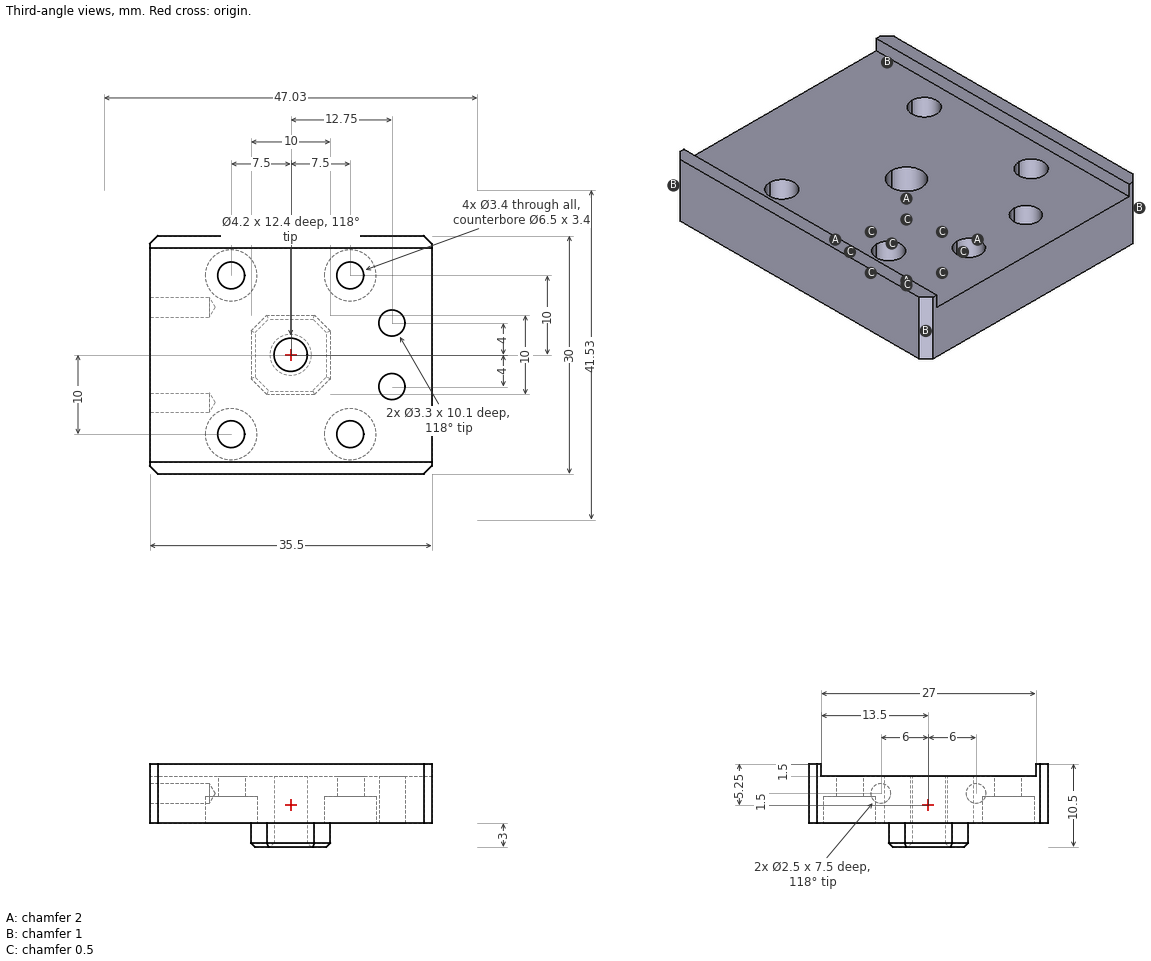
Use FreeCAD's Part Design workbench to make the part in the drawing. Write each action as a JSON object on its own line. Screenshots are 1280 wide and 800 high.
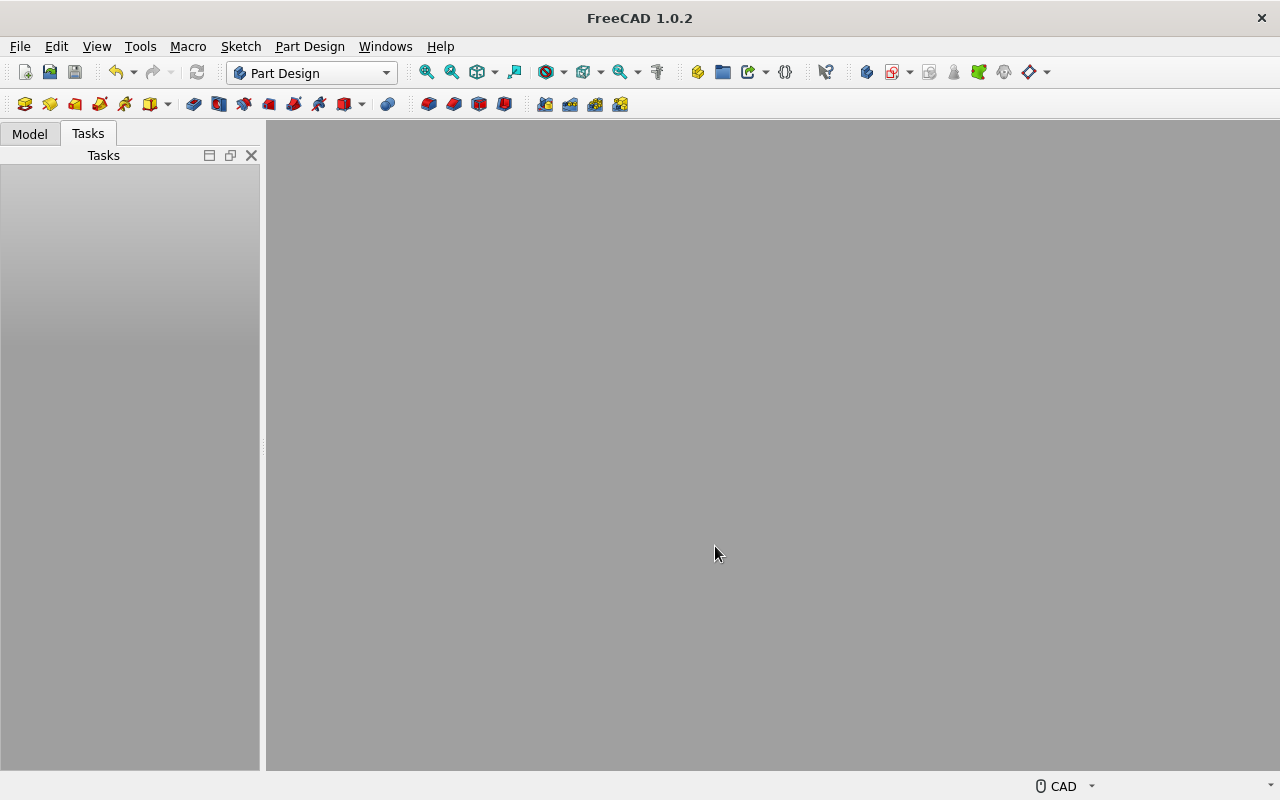
{"action": "key", "text": "ctrl+n"}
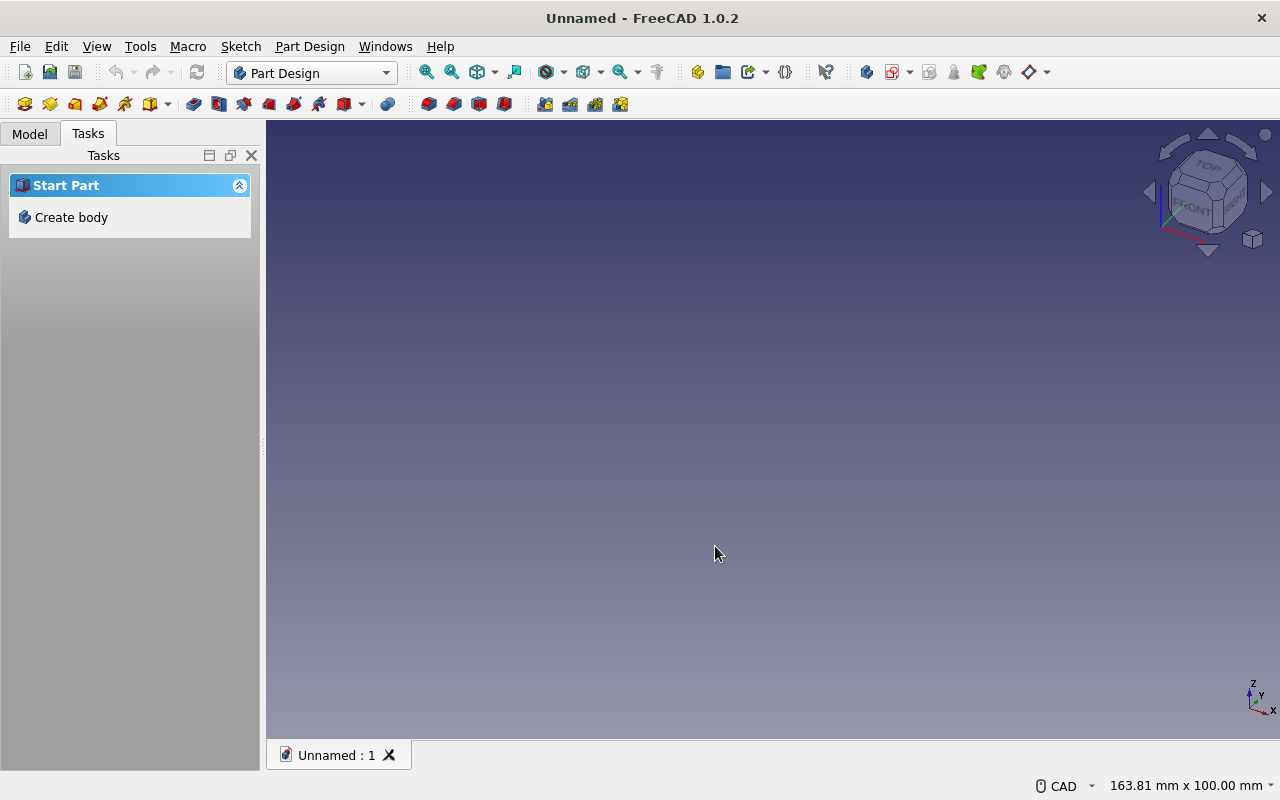
{"action": "left_click", "coordinate": [892, 72]}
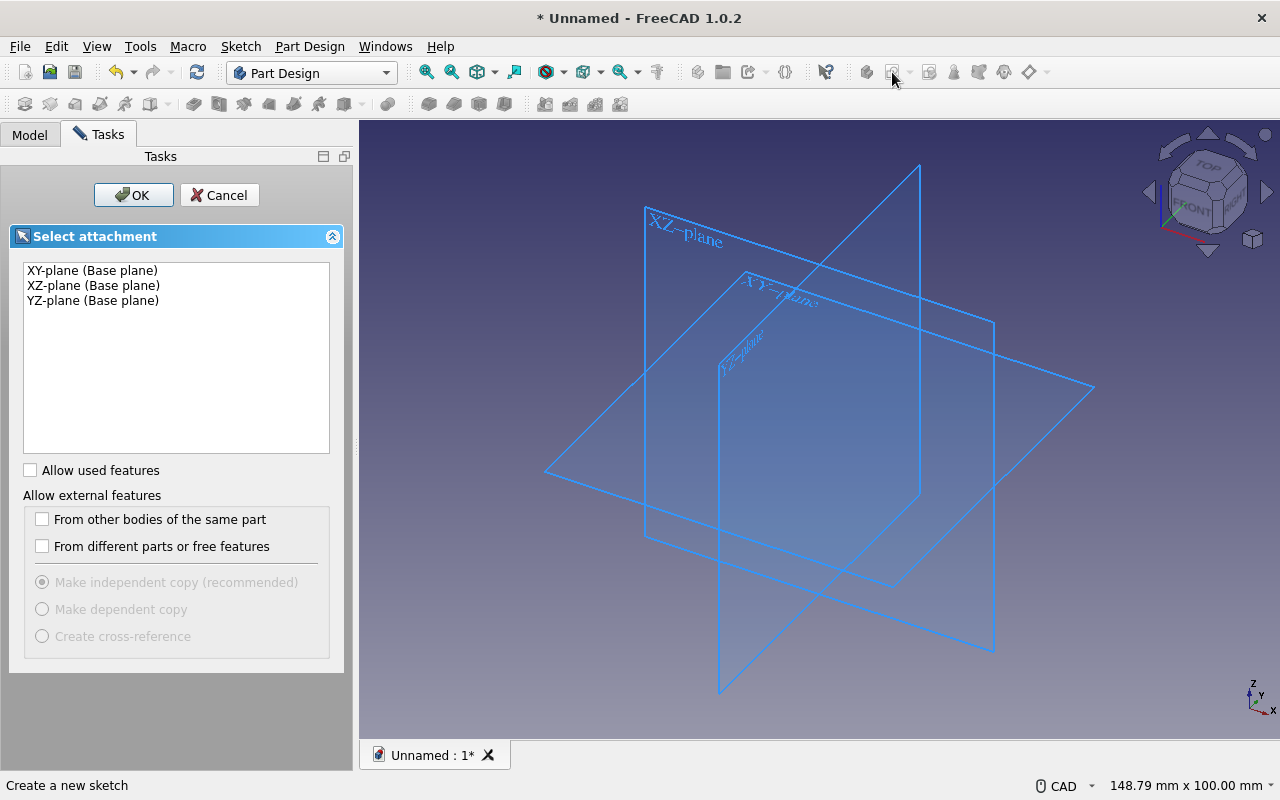
{"action": "left_click", "coordinate": [84, 270]}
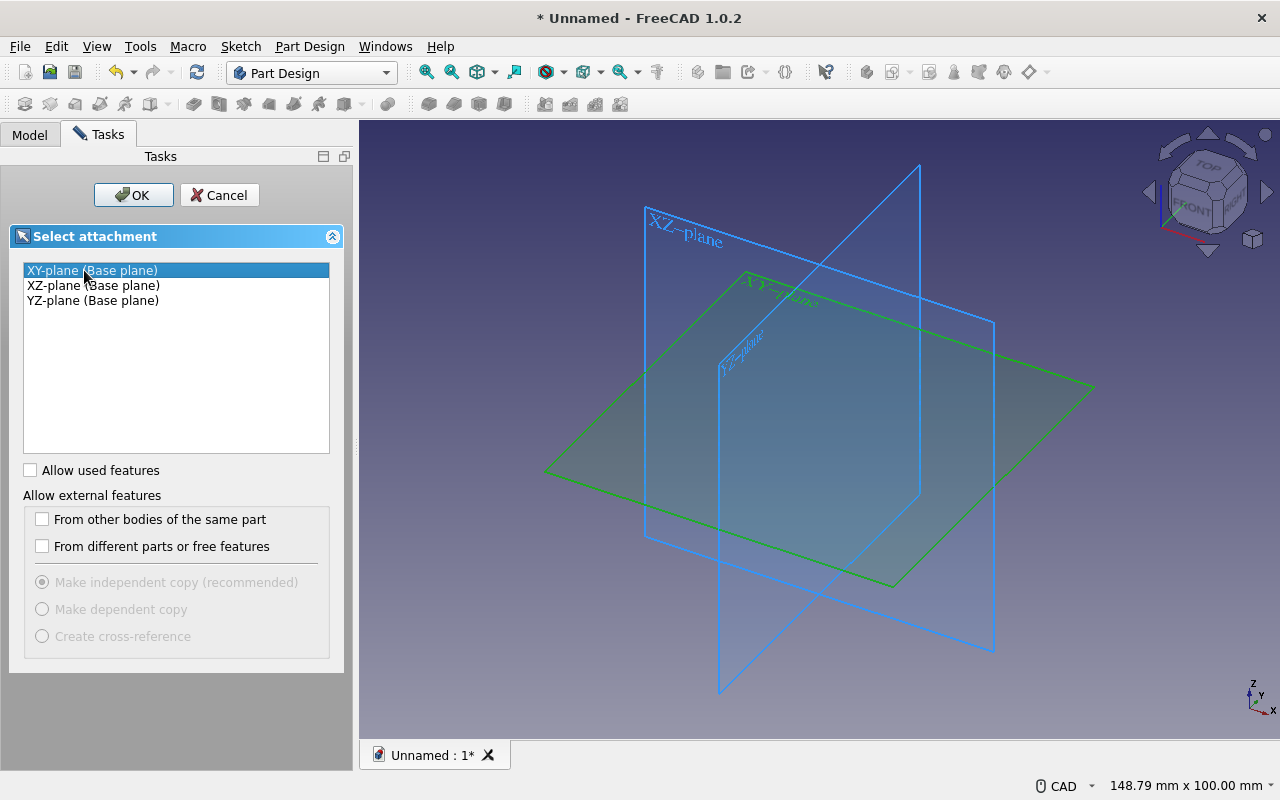
{"action": "left_click", "coordinate": [134, 195]}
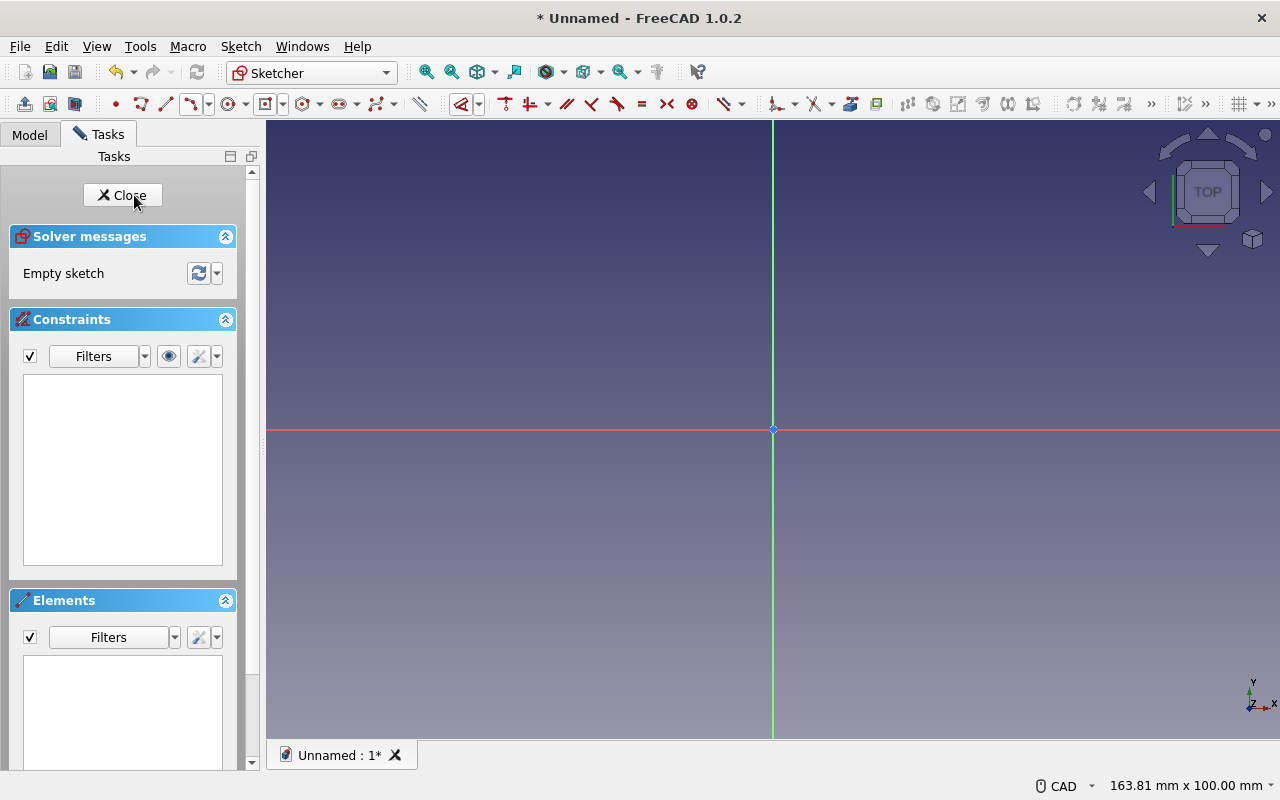
{"action": "scroll", "coordinate": [829, 430], "scroll_direction": "up", "scroll_amount": 4}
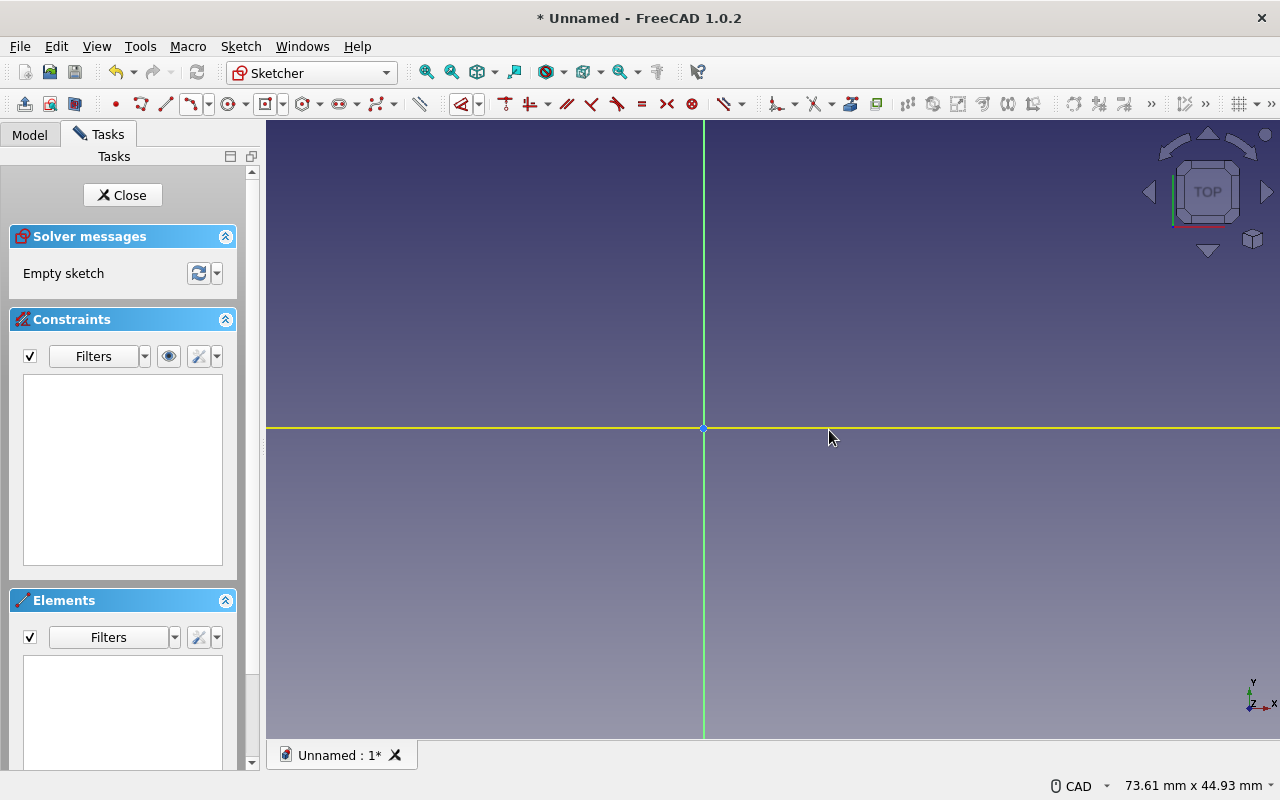
{"action": "key", "text": "g v"}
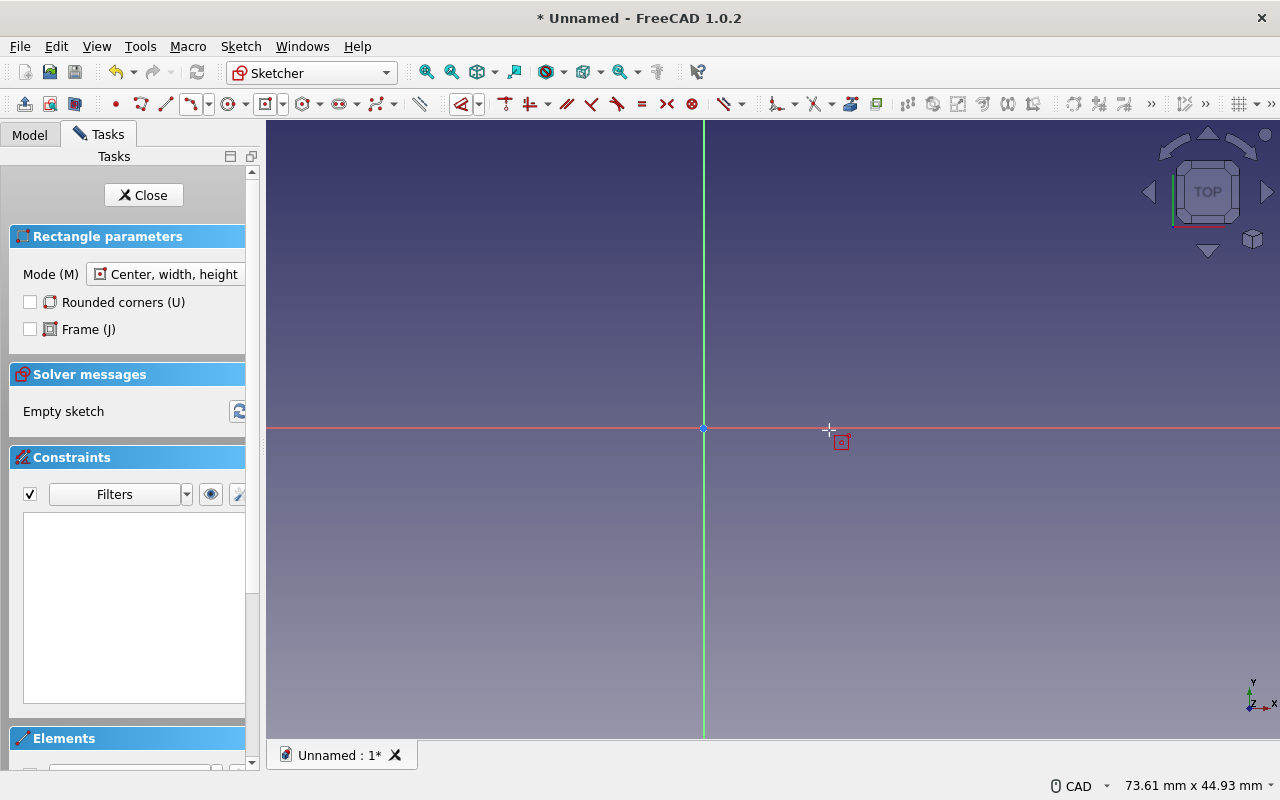
{"action": "left_click", "coordinate": [704, 428]}
{"action": "left_click", "coordinate": [948, 222]}
{"action": "key", "text": "Escape"}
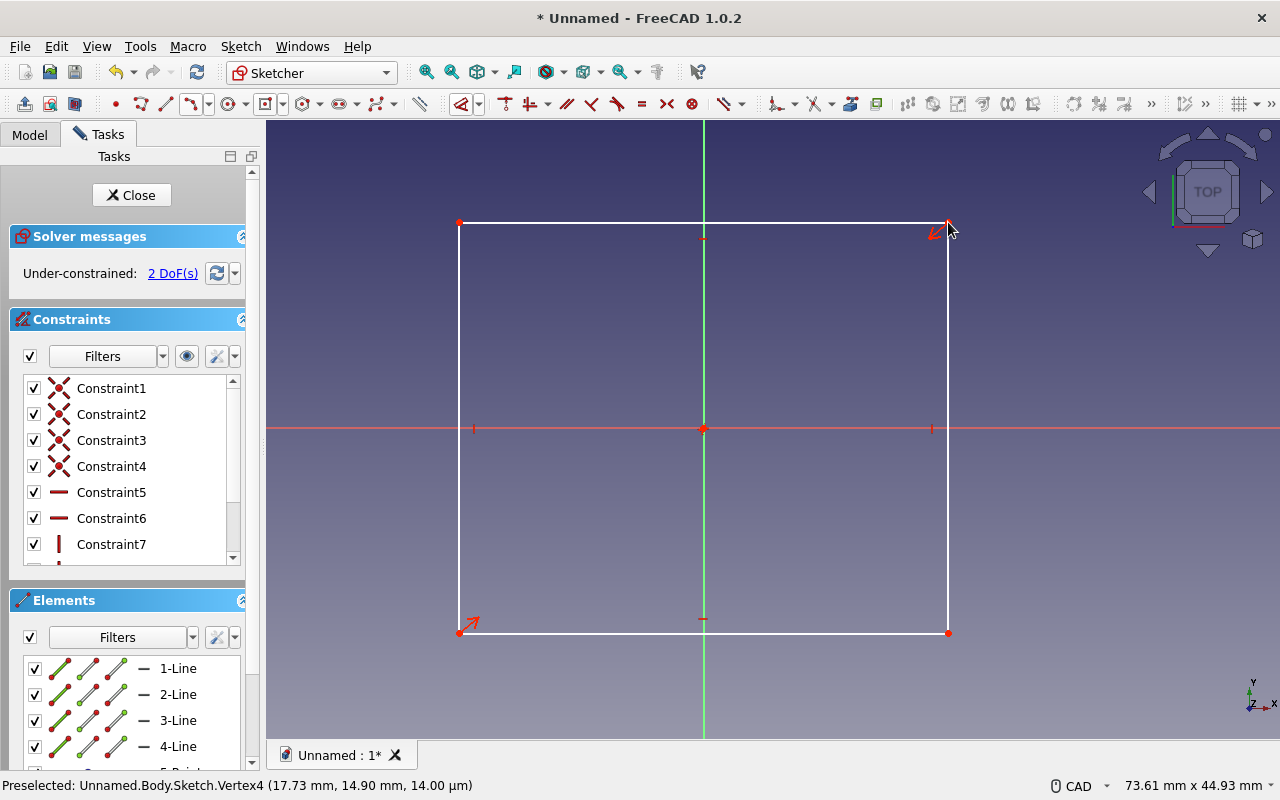
{"action": "key", "text": "d"}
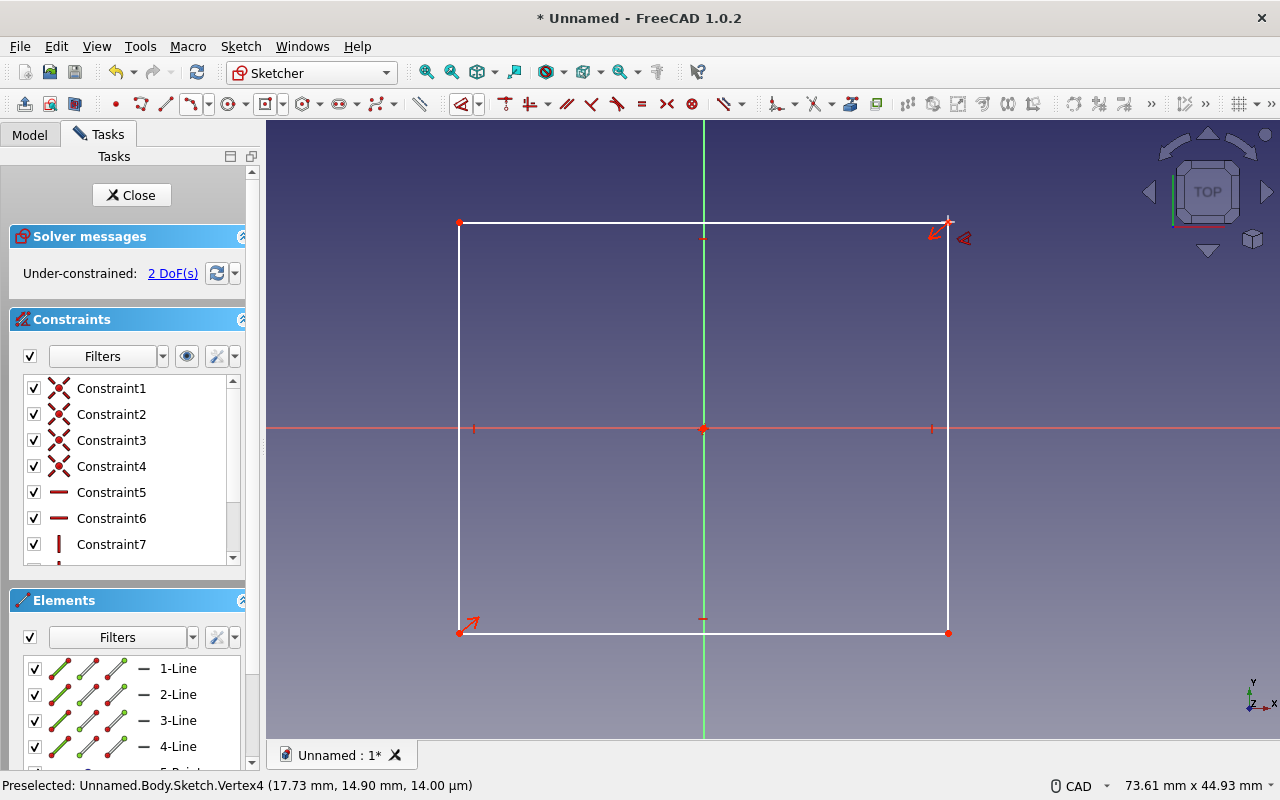
{"action": "left_click", "coordinate": [948, 510]}
{"action": "left_click", "coordinate": [982, 334]}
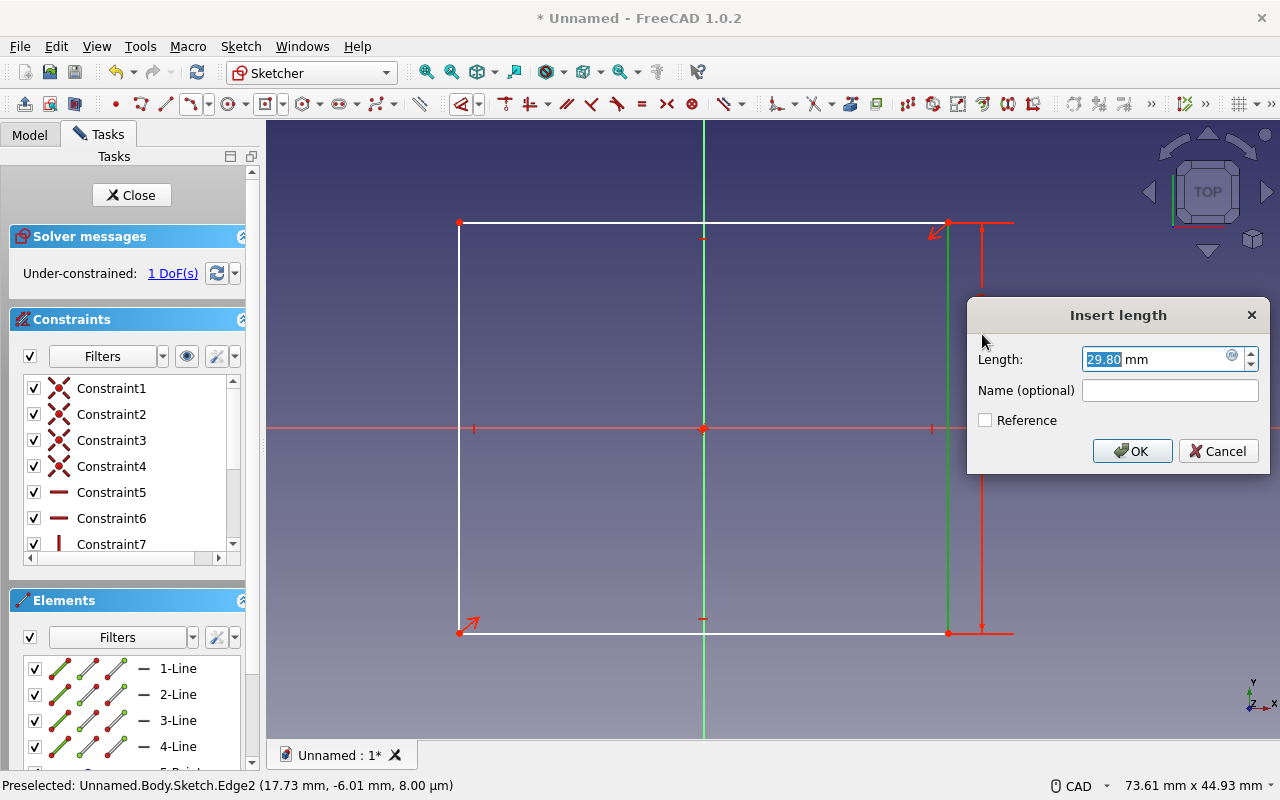
{"action": "type", "text": "30"}
{"action": "key", "text": "Return"}